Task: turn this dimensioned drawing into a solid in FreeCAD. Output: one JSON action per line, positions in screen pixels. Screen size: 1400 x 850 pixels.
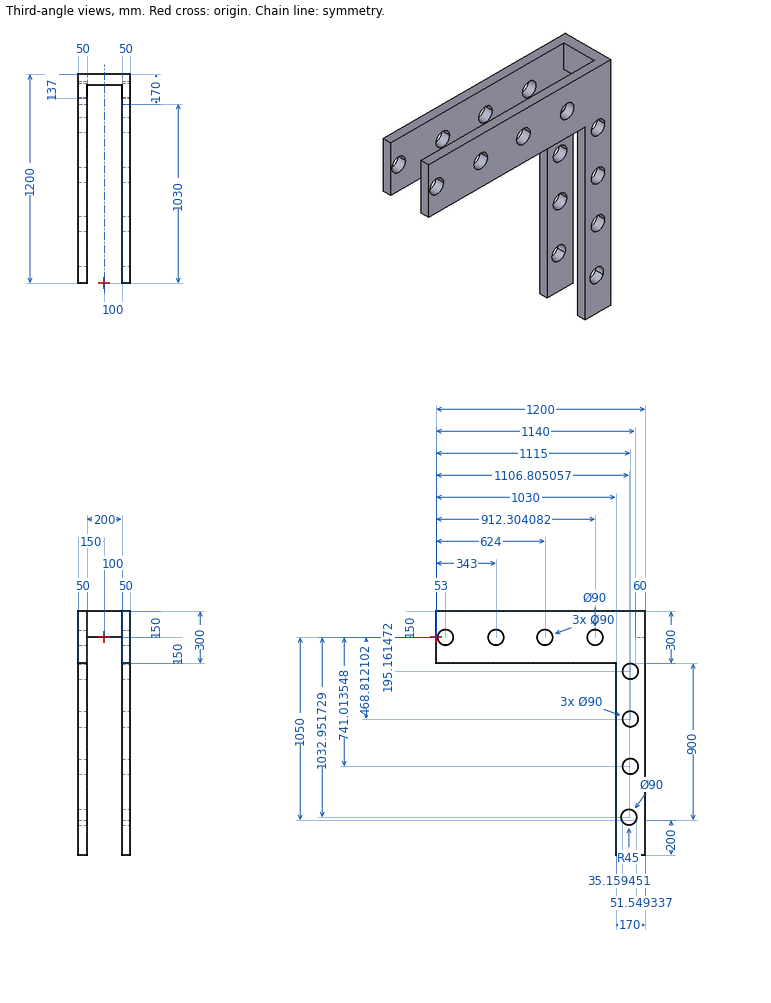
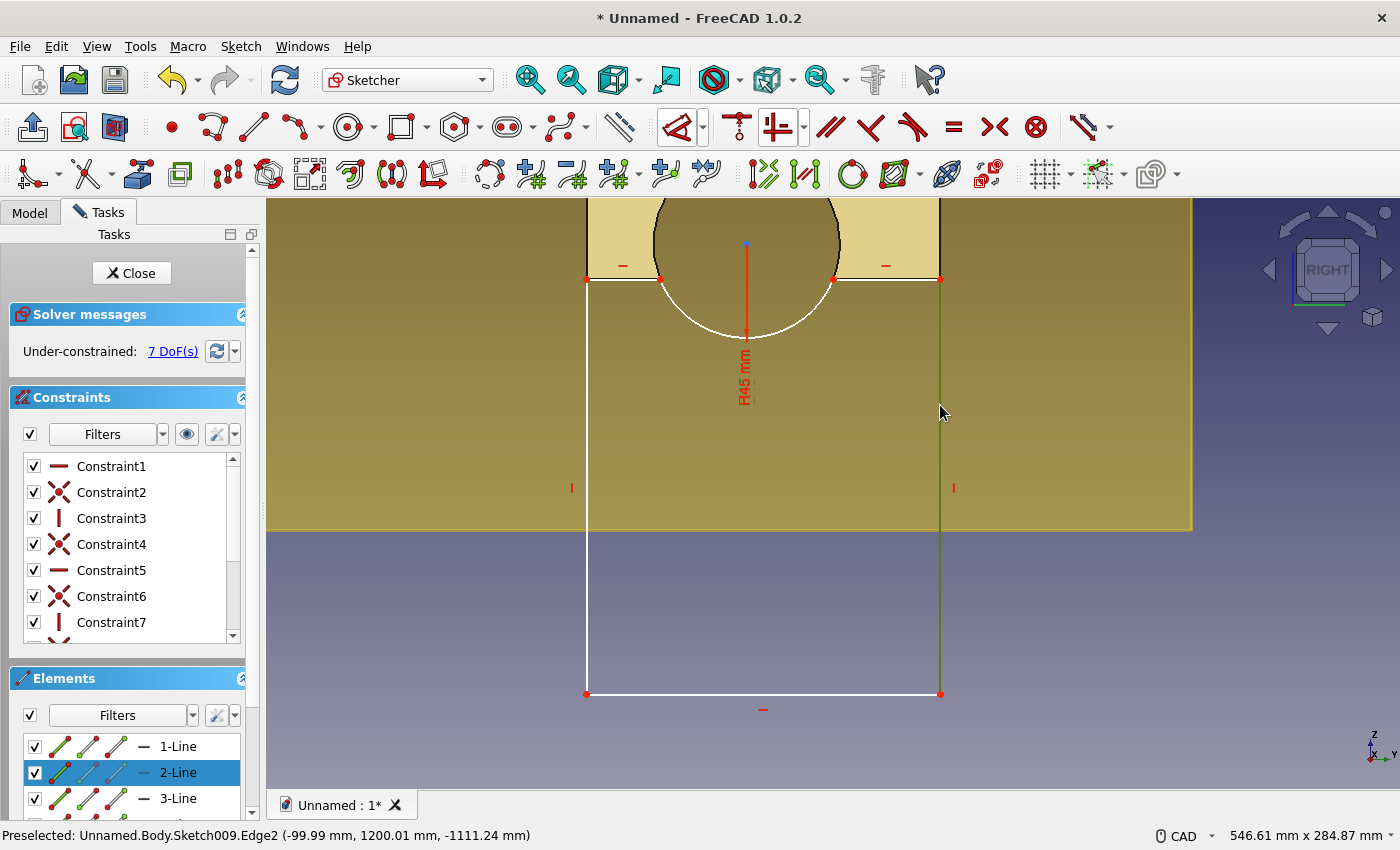
{"action": "left_click", "coordinate": [702, 128]}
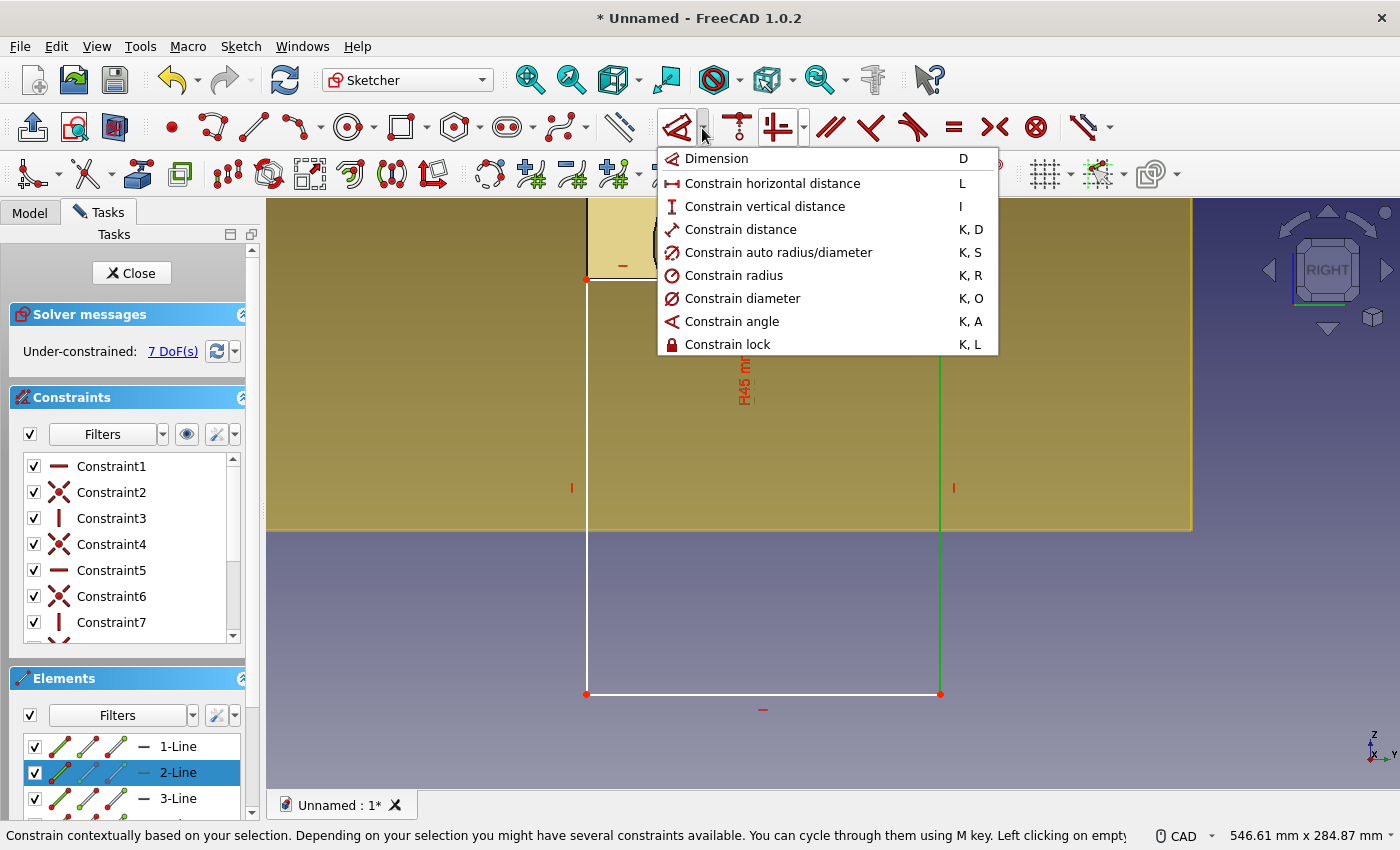
{"action": "left_click", "coordinate": [828, 206]}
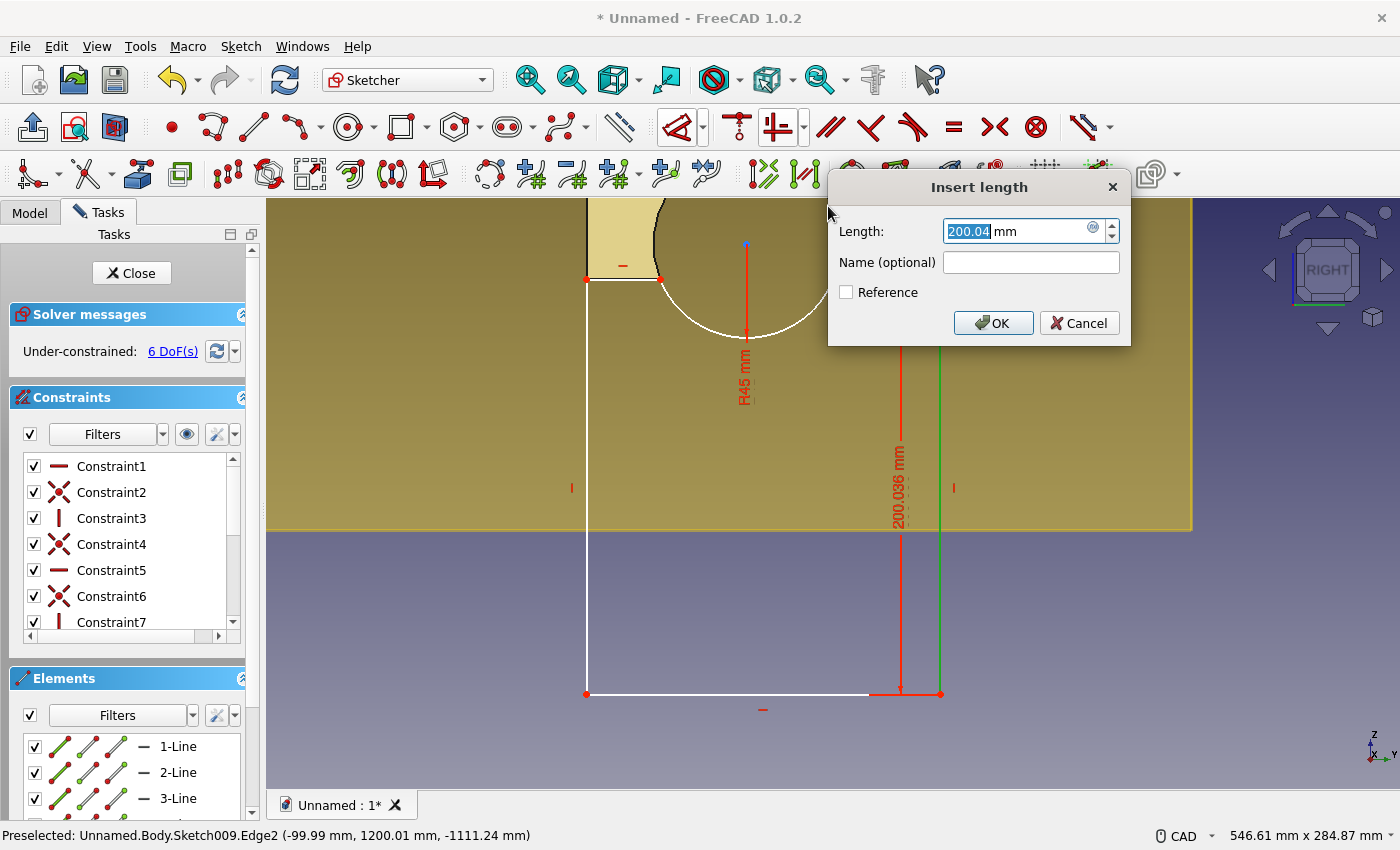
{"action": "type", "text": "200"}
{"action": "key", "text": "Return"}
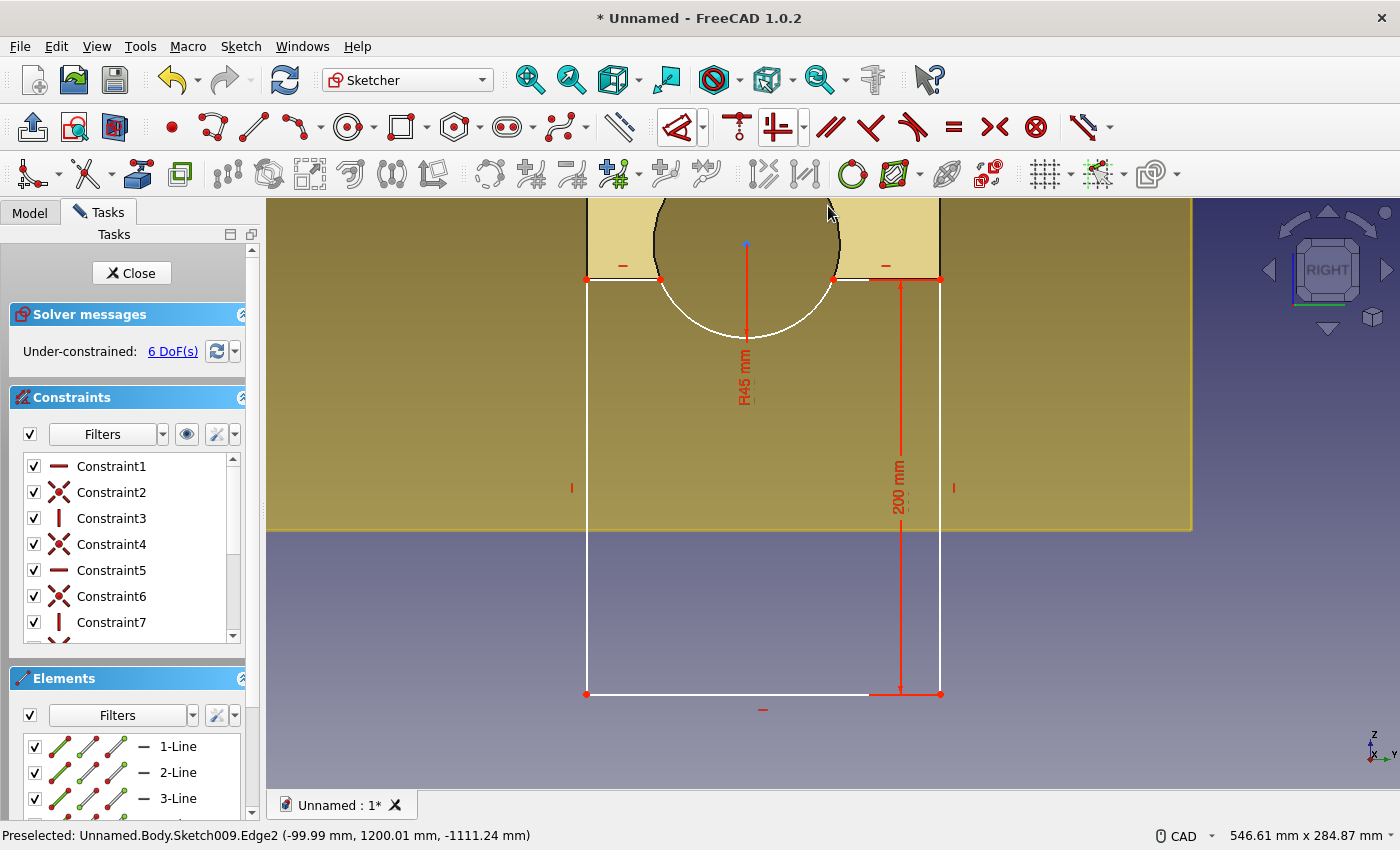
{"action": "left_click", "coordinate": [834, 695]}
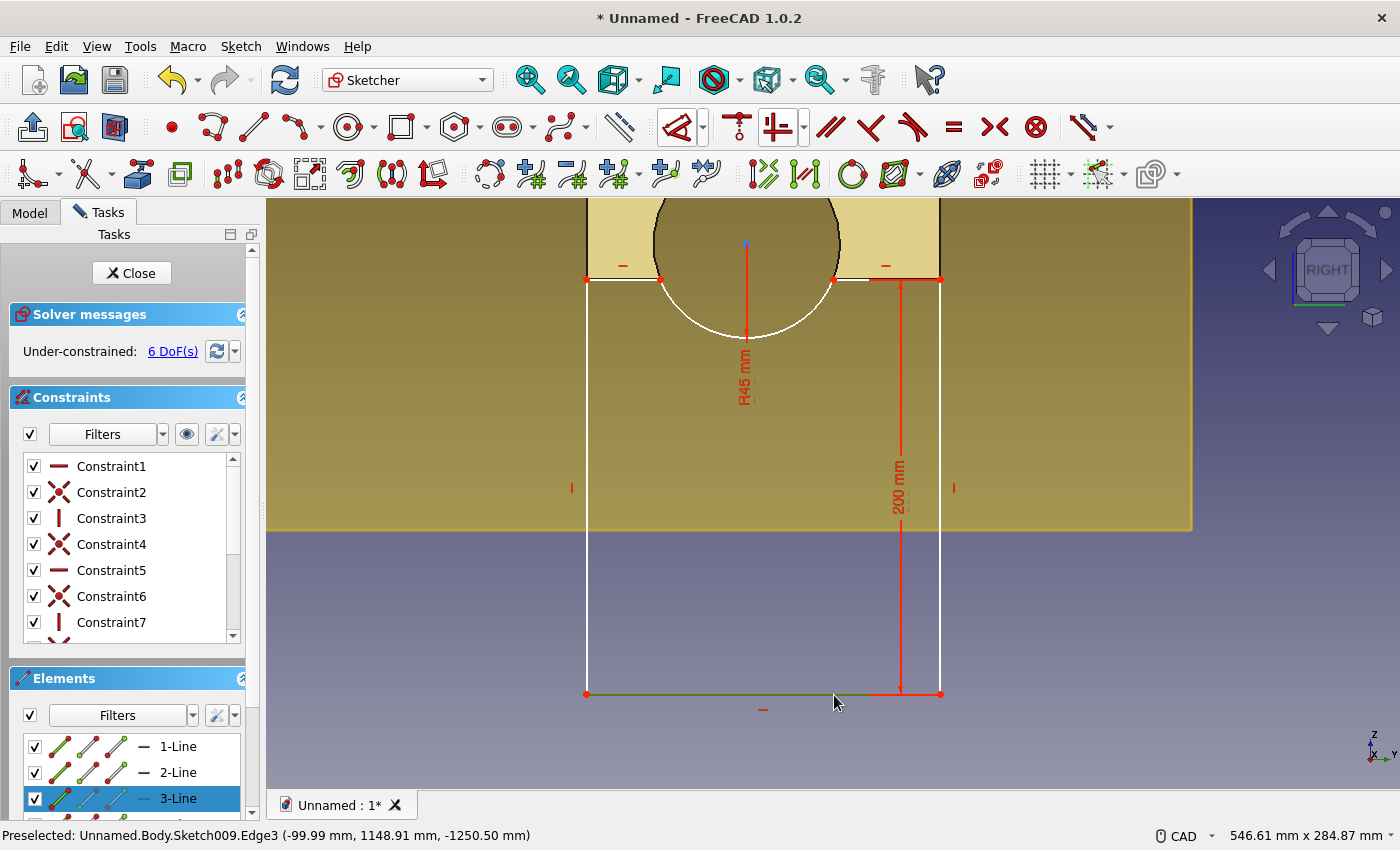
{"action": "left_click", "coordinate": [702, 128]}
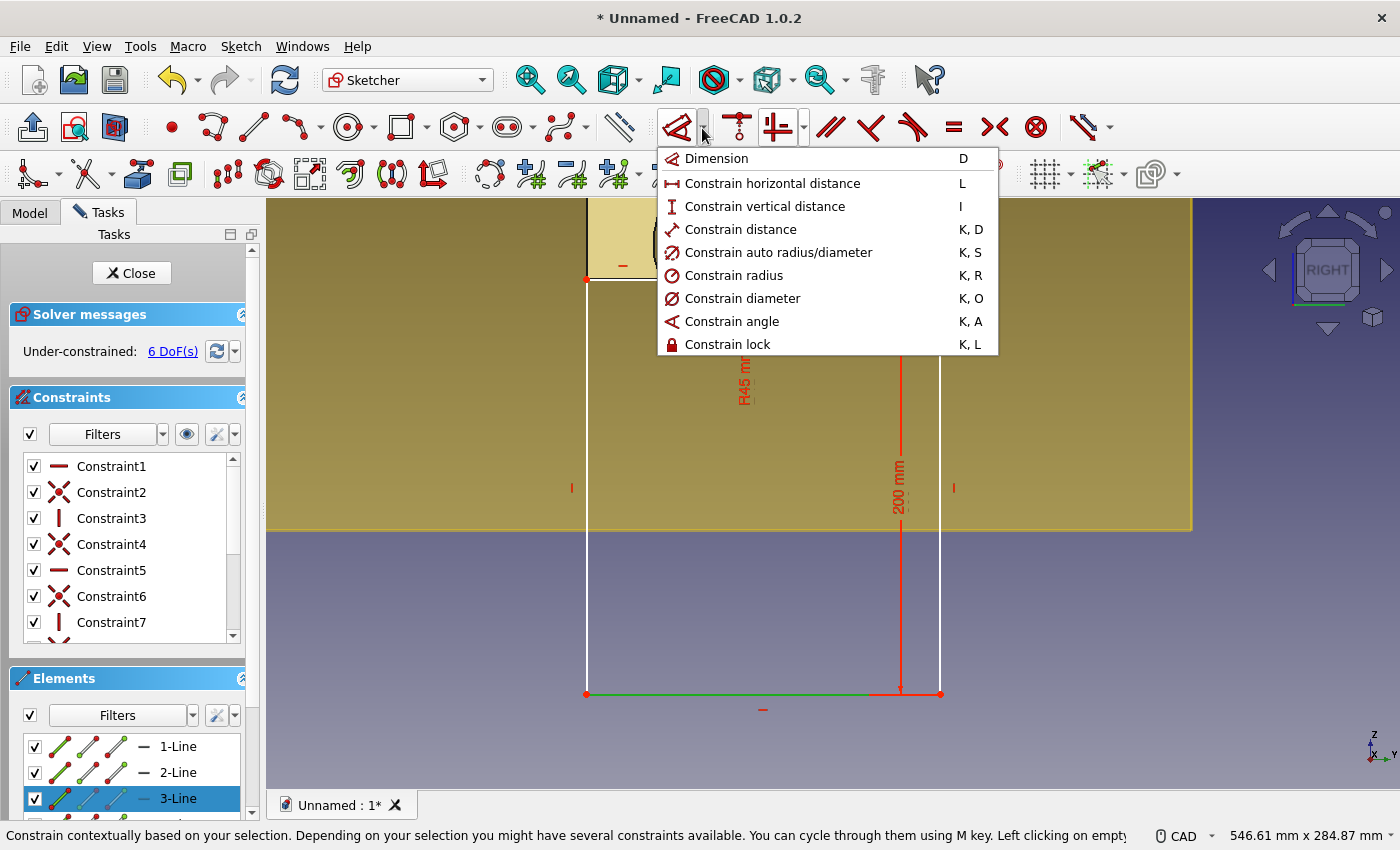
{"action": "left_click", "coordinate": [828, 184]}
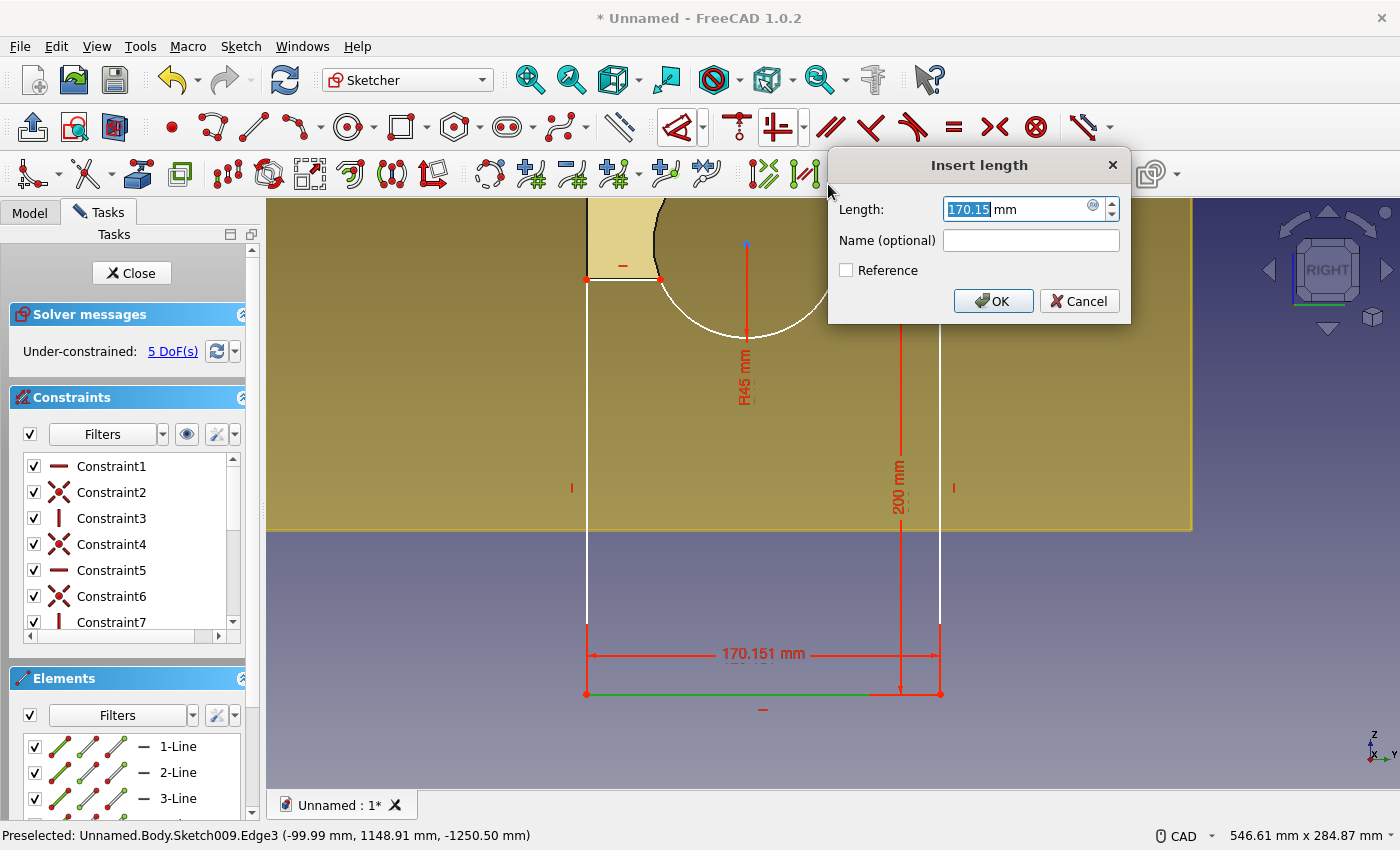
{"action": "type", "text": "170"}
{"action": "key", "text": "Return"}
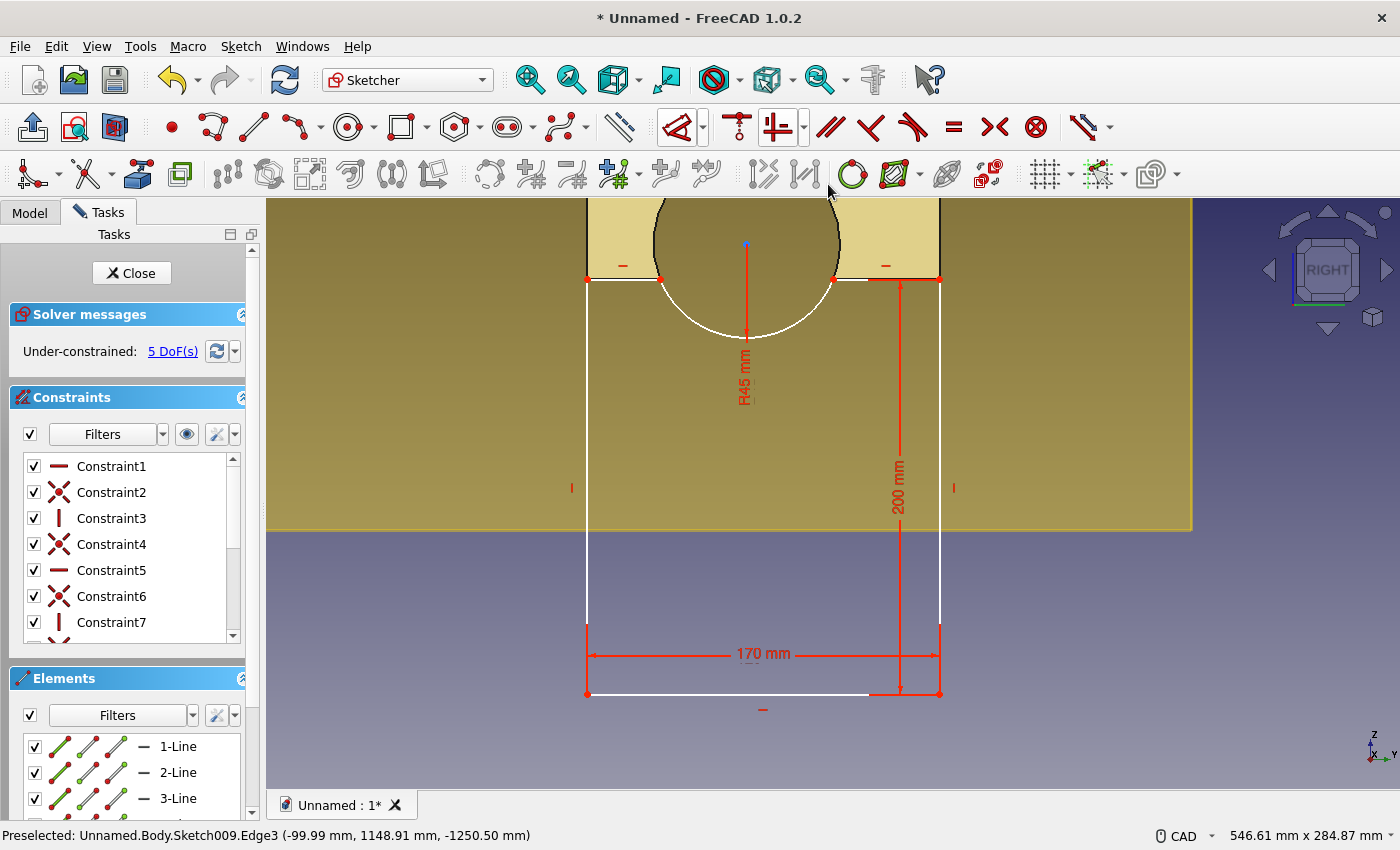
{"action": "left_click", "coordinate": [587, 570]}